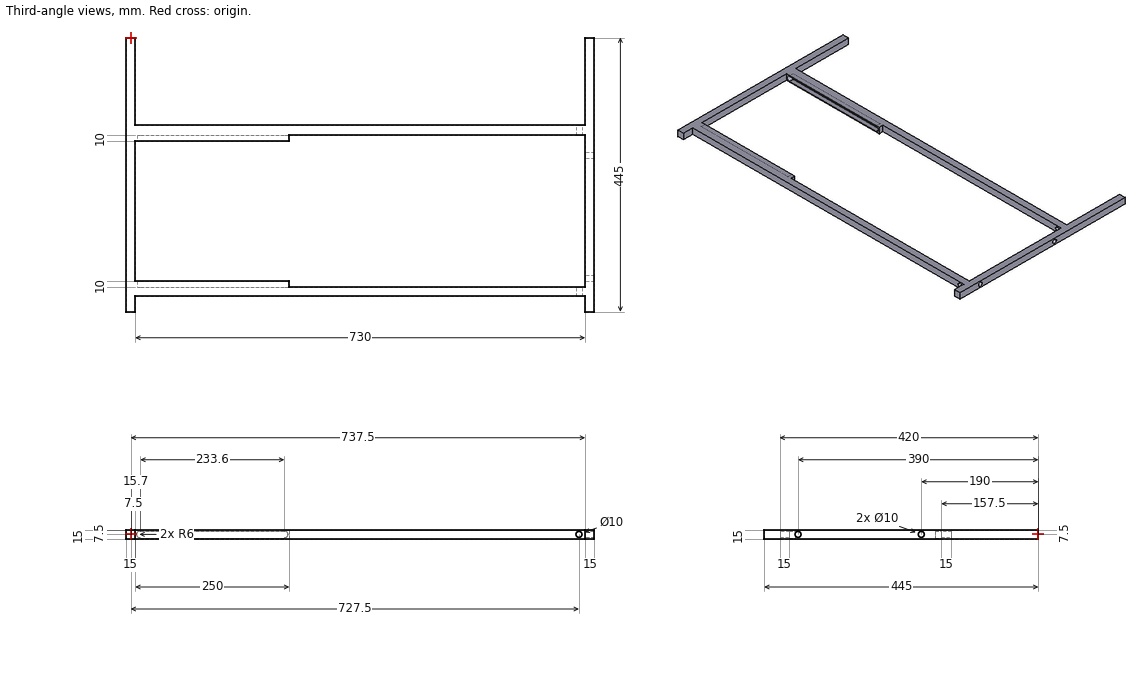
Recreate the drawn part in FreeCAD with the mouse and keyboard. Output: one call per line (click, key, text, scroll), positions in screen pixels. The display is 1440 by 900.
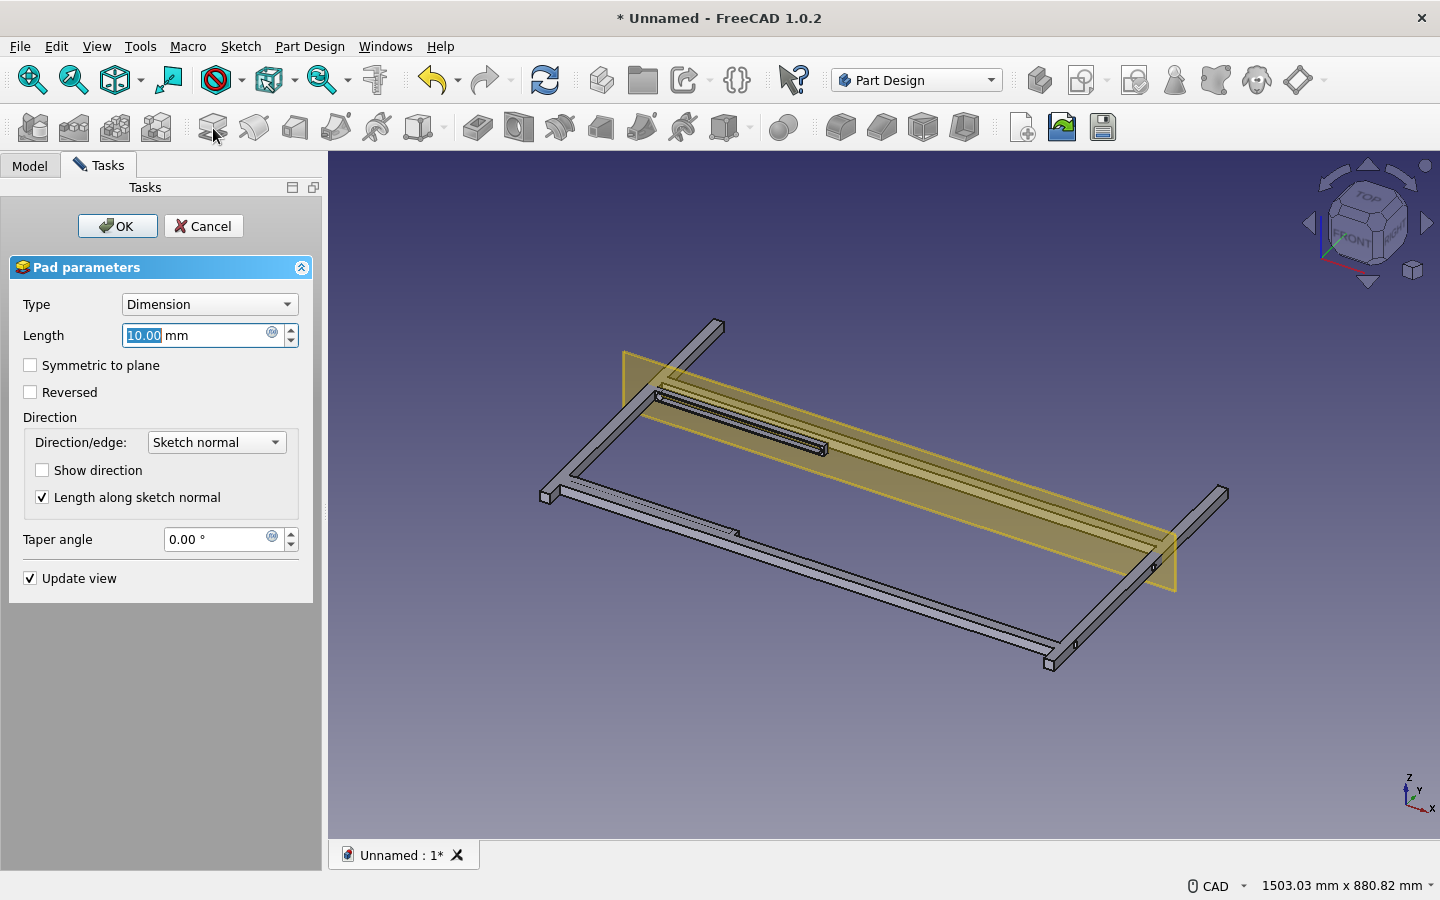
text(10)
key(Tab)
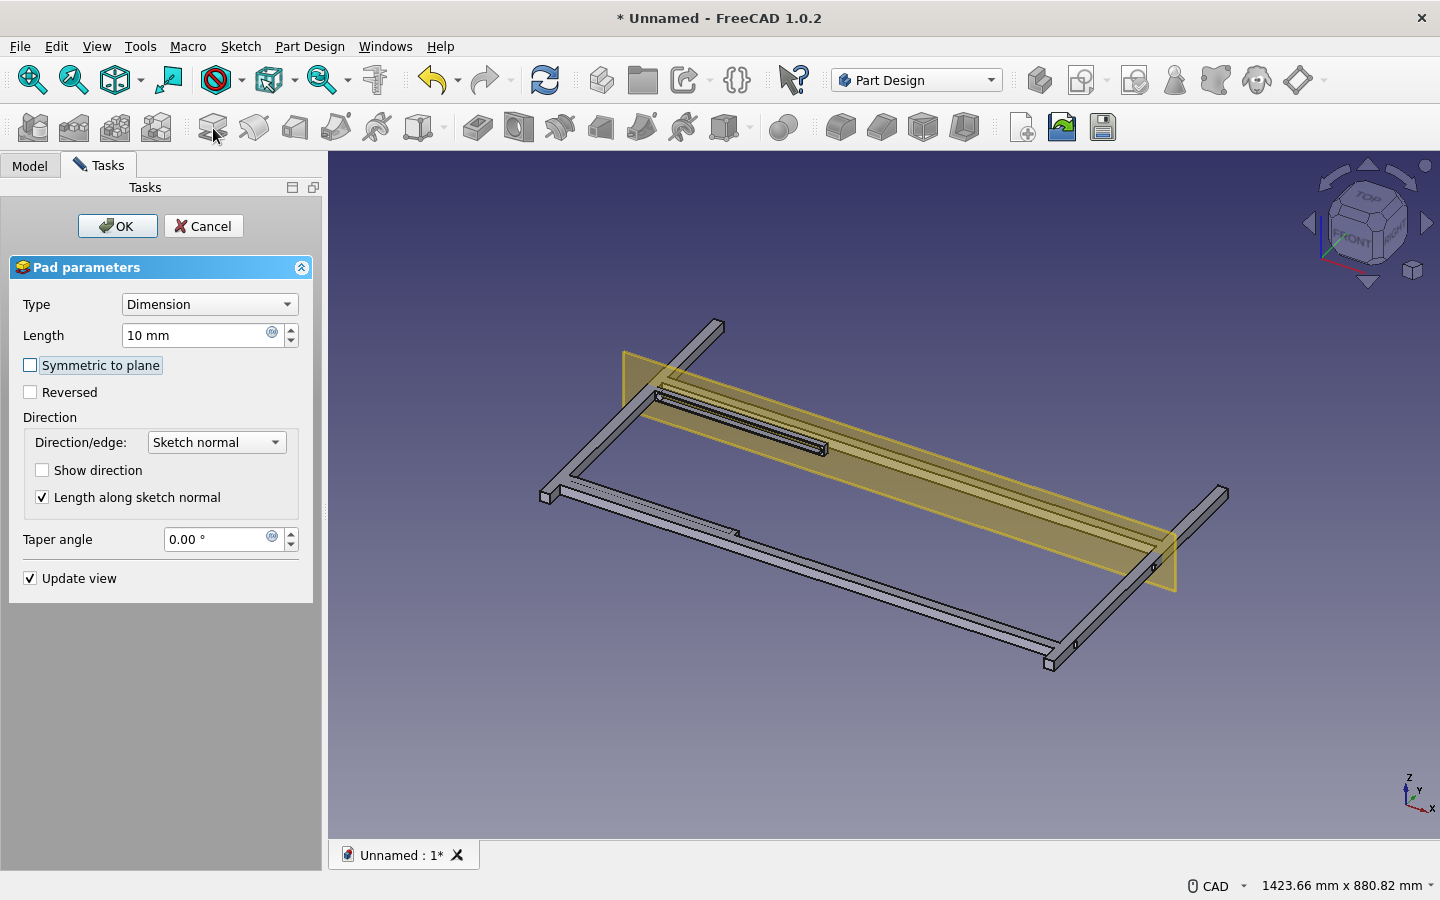
click(31, 392)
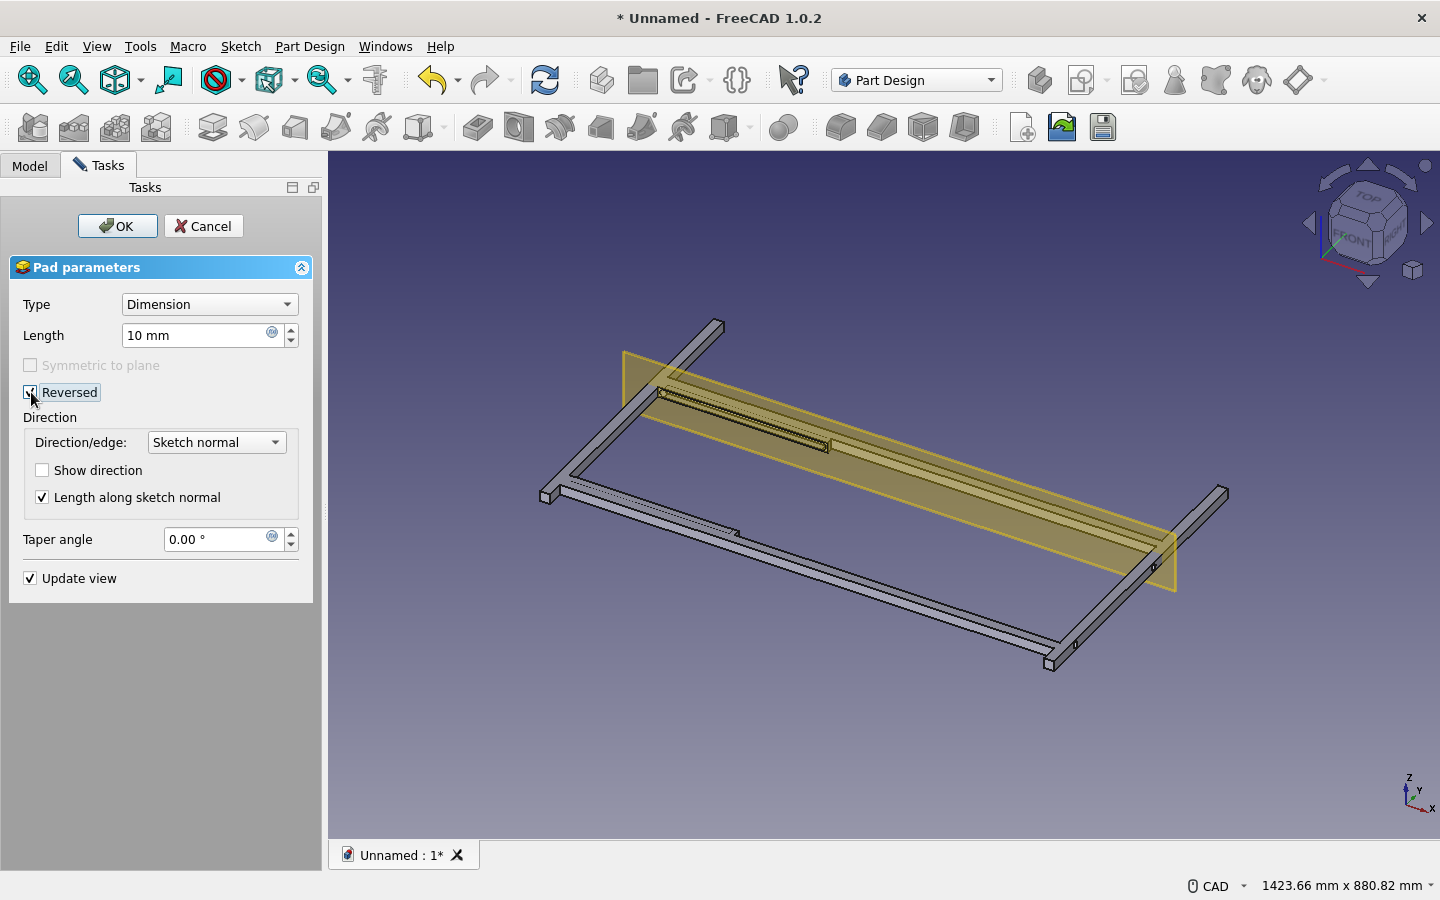
click(118, 226)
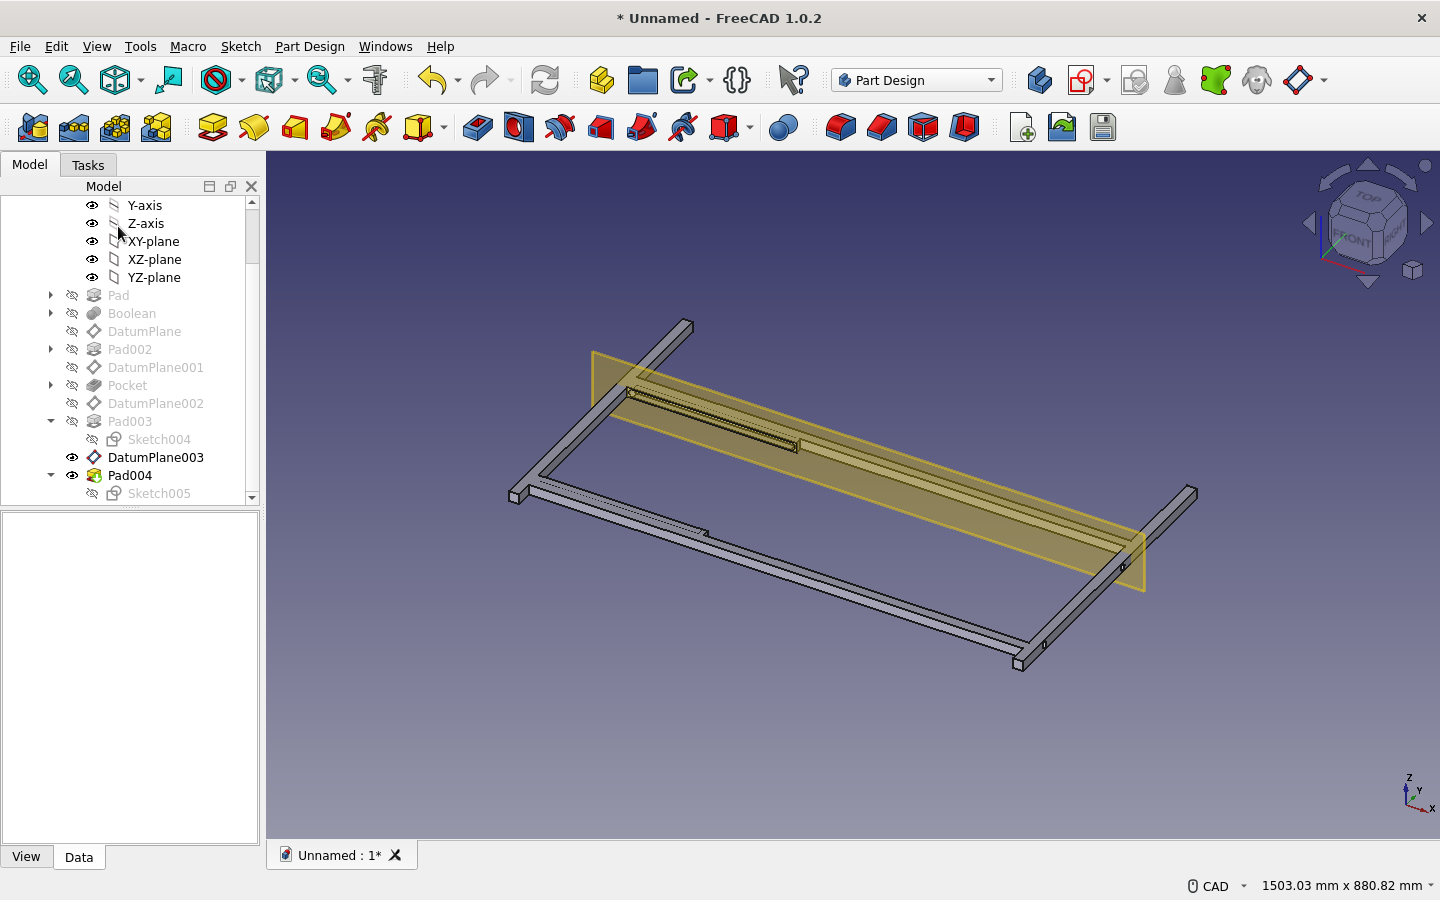
click(117, 457)
key(space)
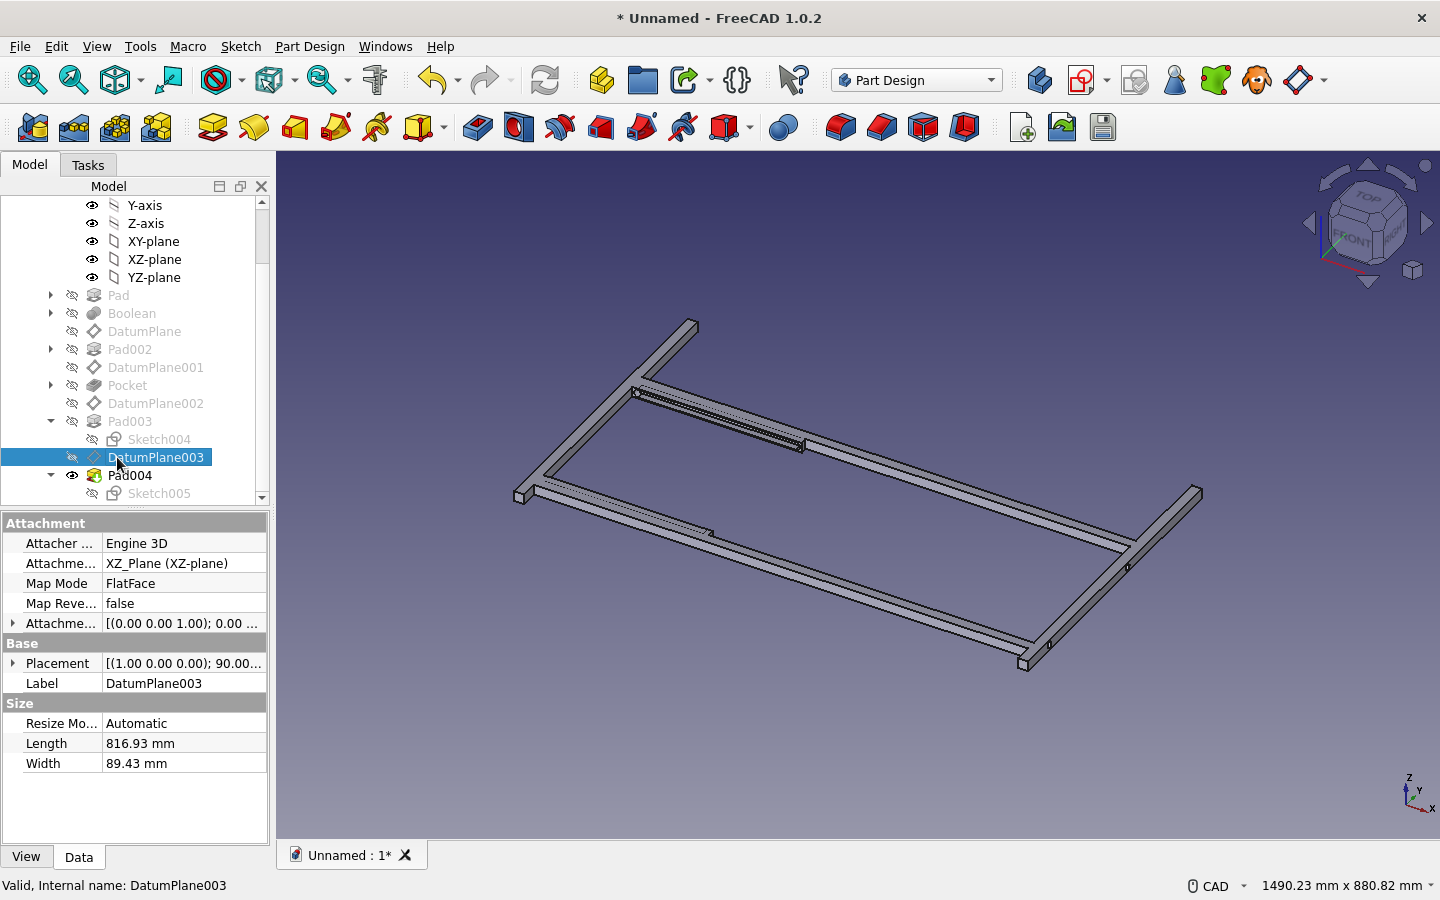
key(4)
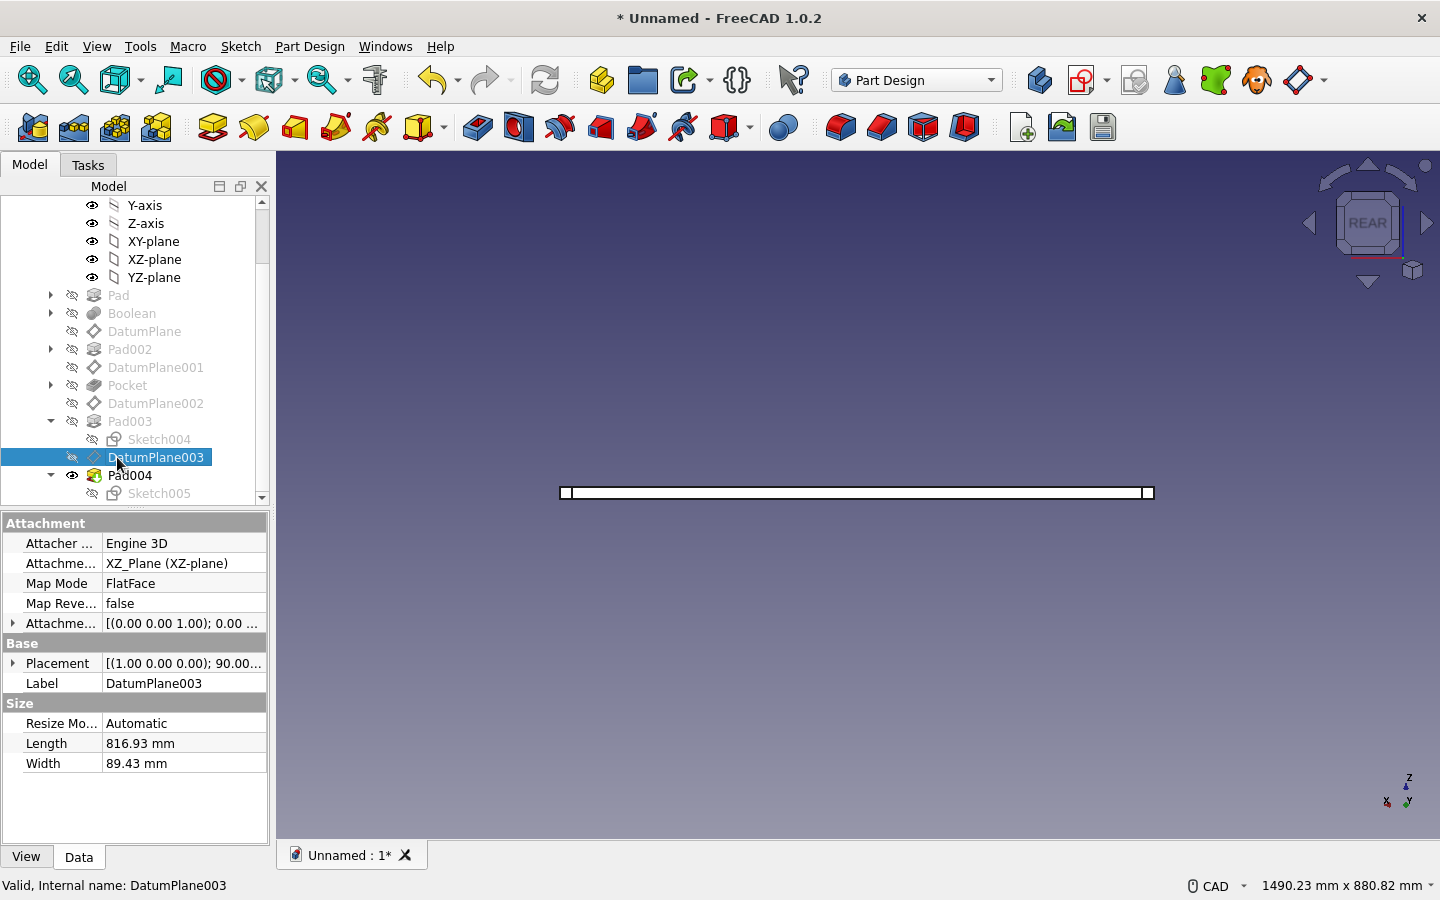
scroll(613, 492, up, 4)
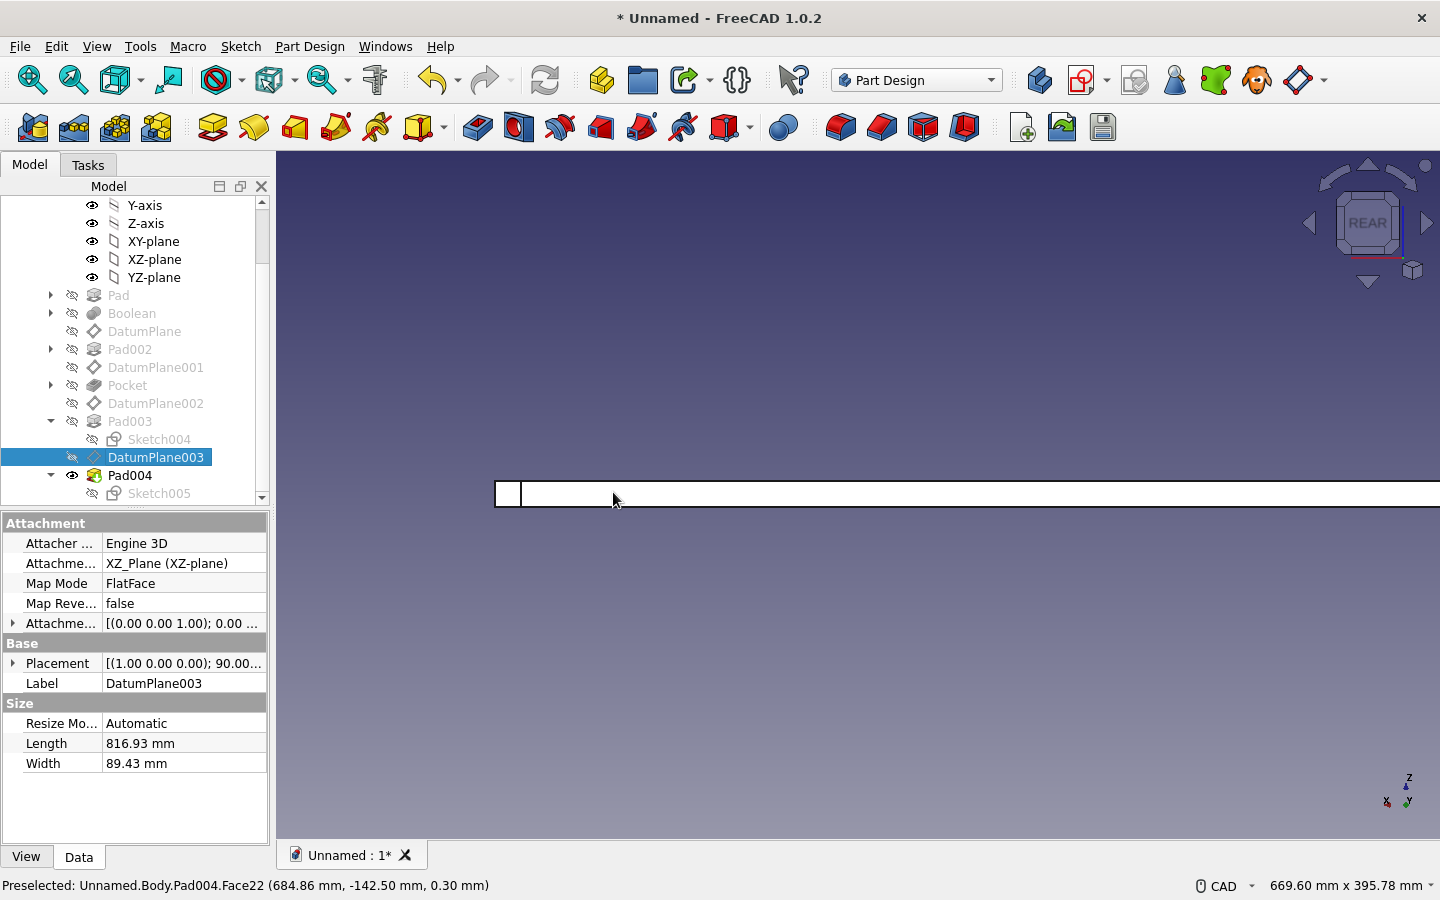
click(612, 493)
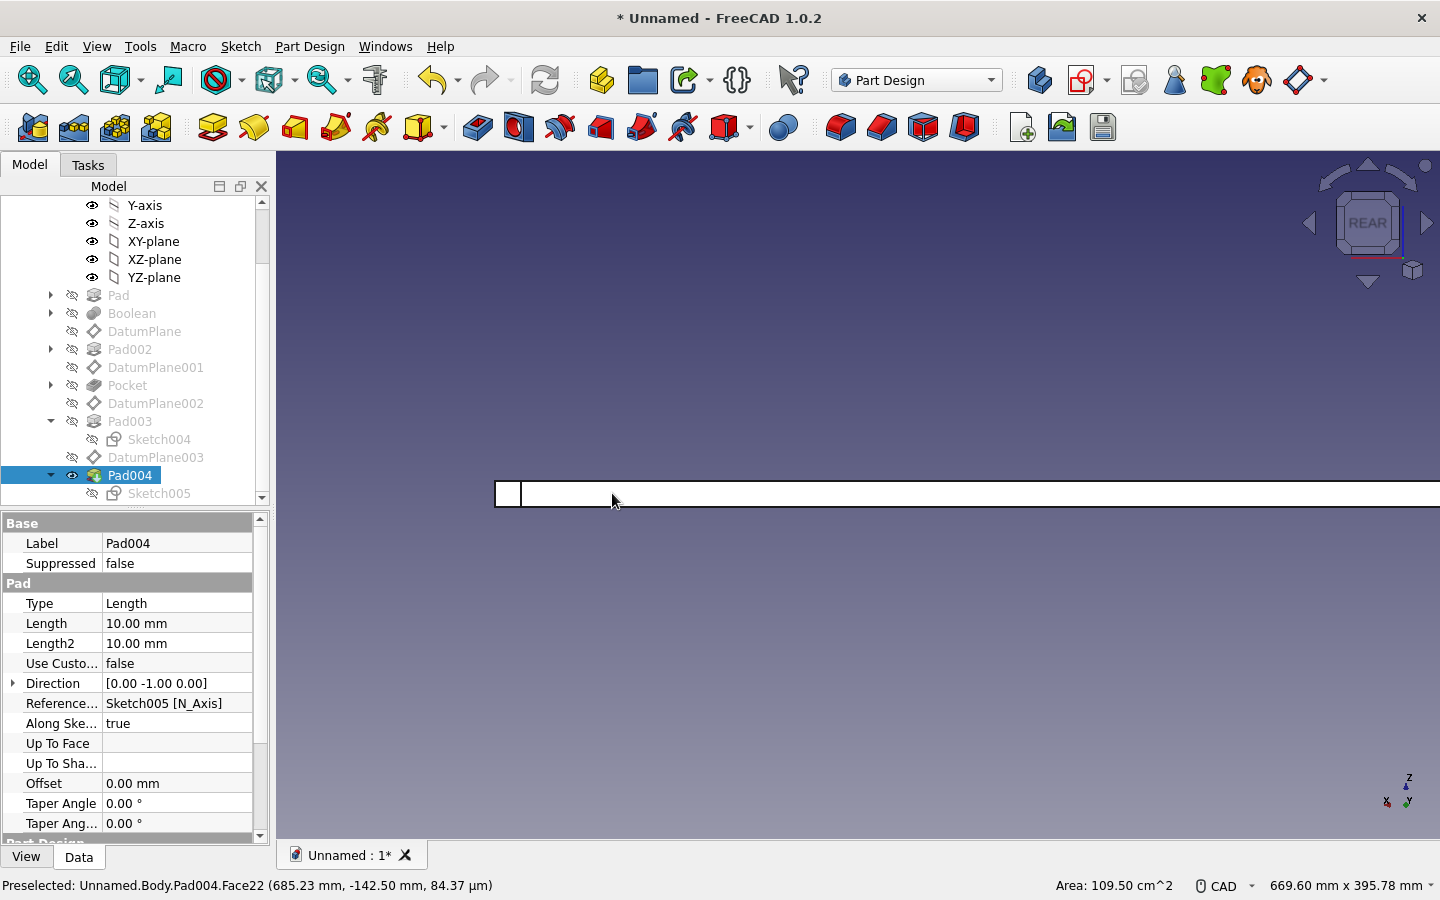
click(1080, 80)